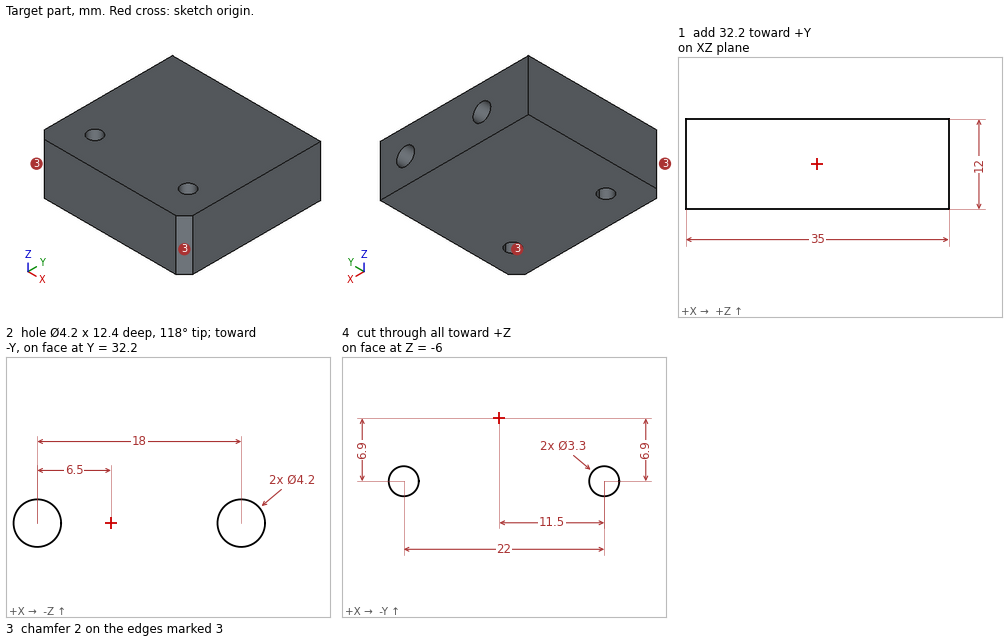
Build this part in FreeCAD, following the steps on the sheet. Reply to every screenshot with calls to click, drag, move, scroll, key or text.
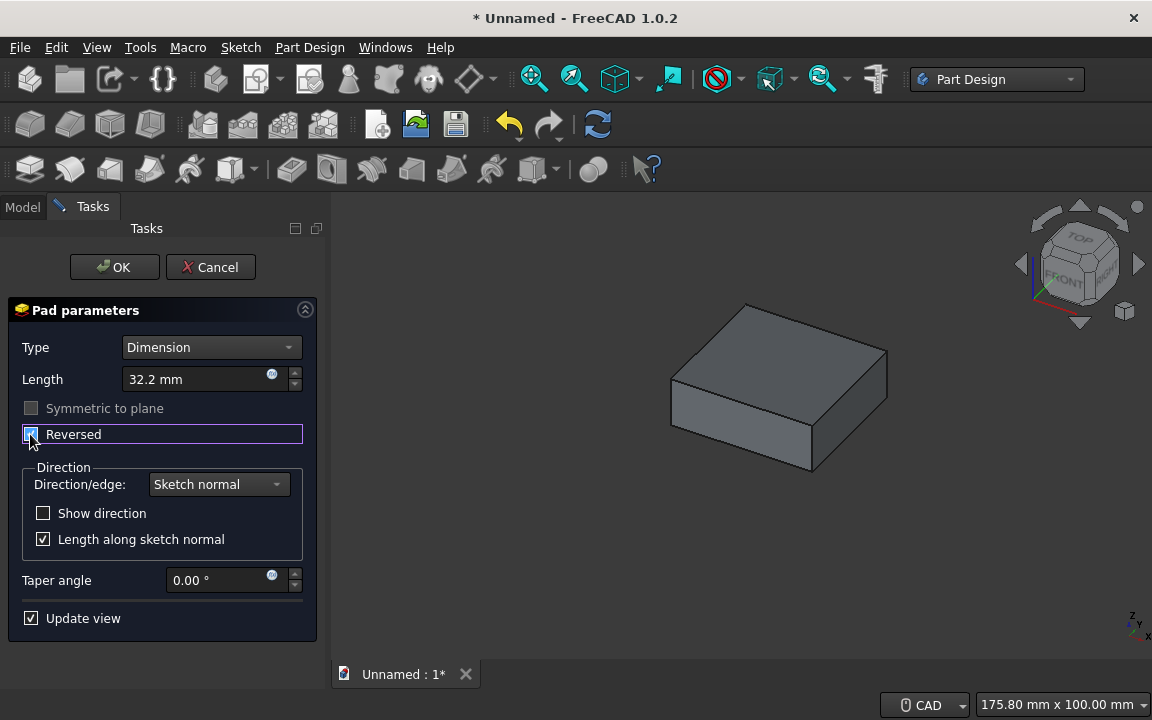
click(115, 267)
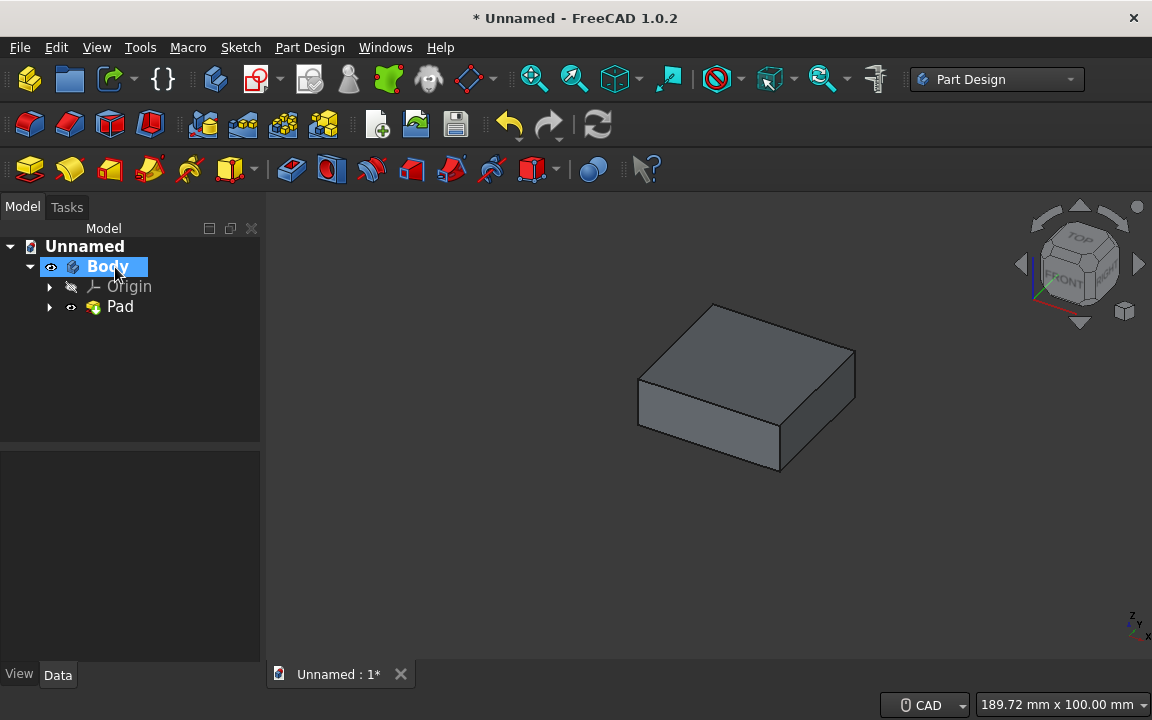
key(v)
key(f)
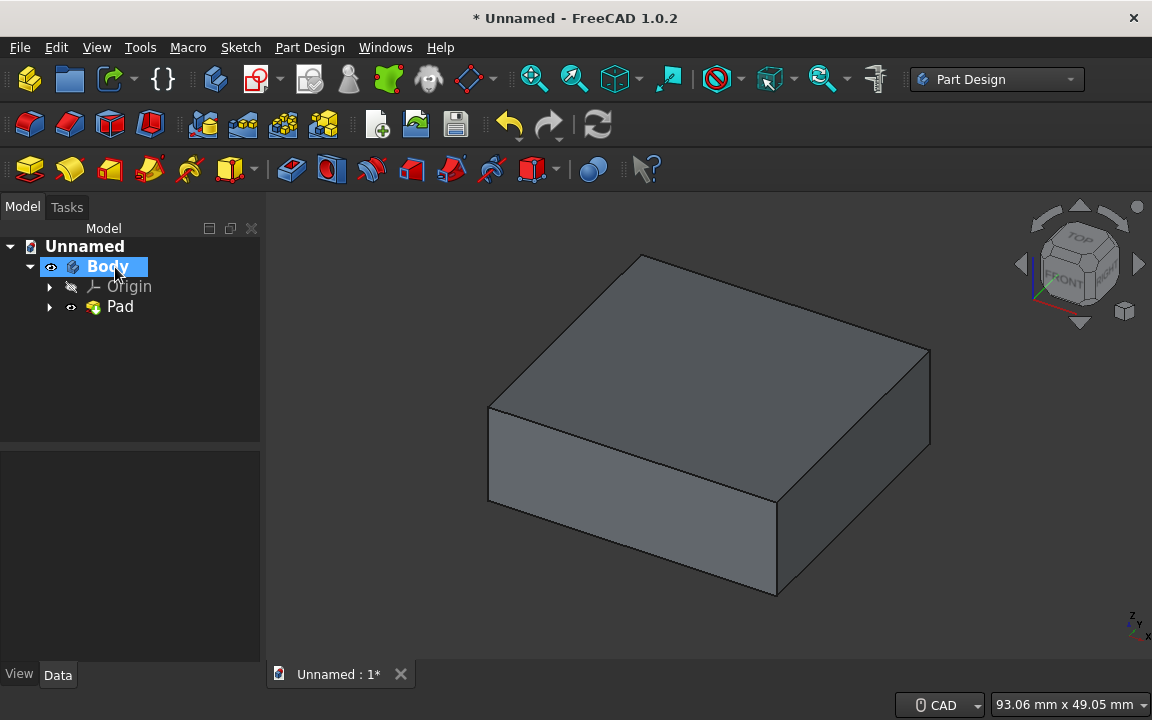
key(4)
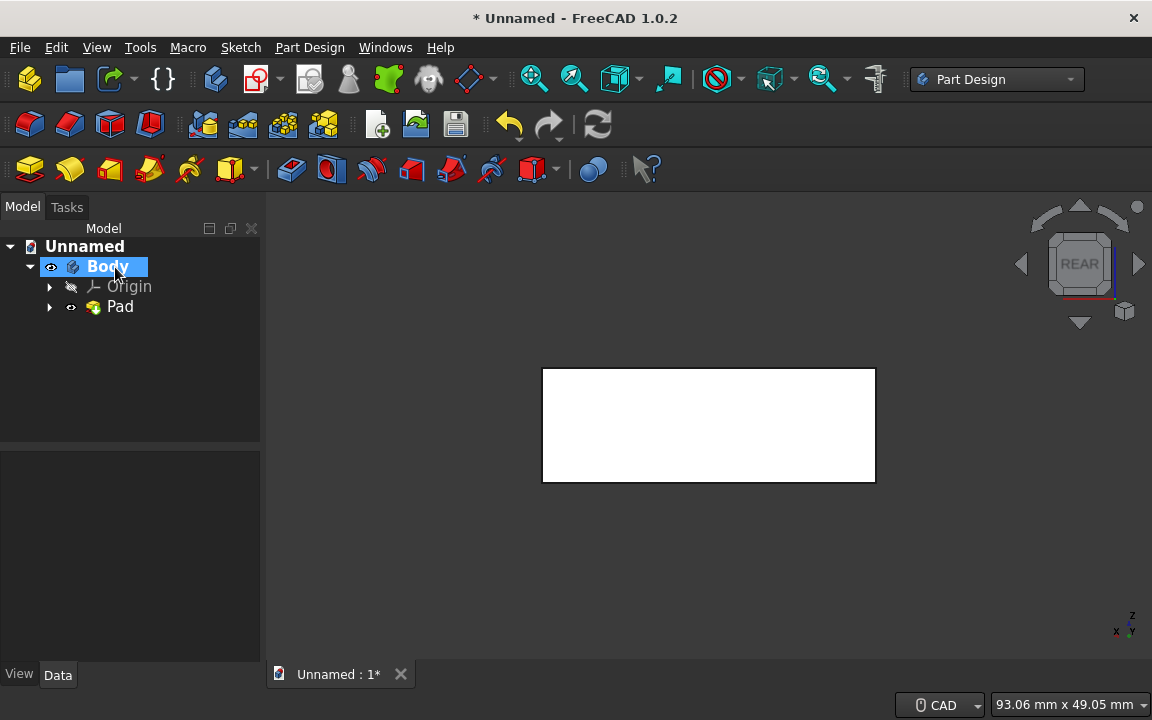
click(536, 80)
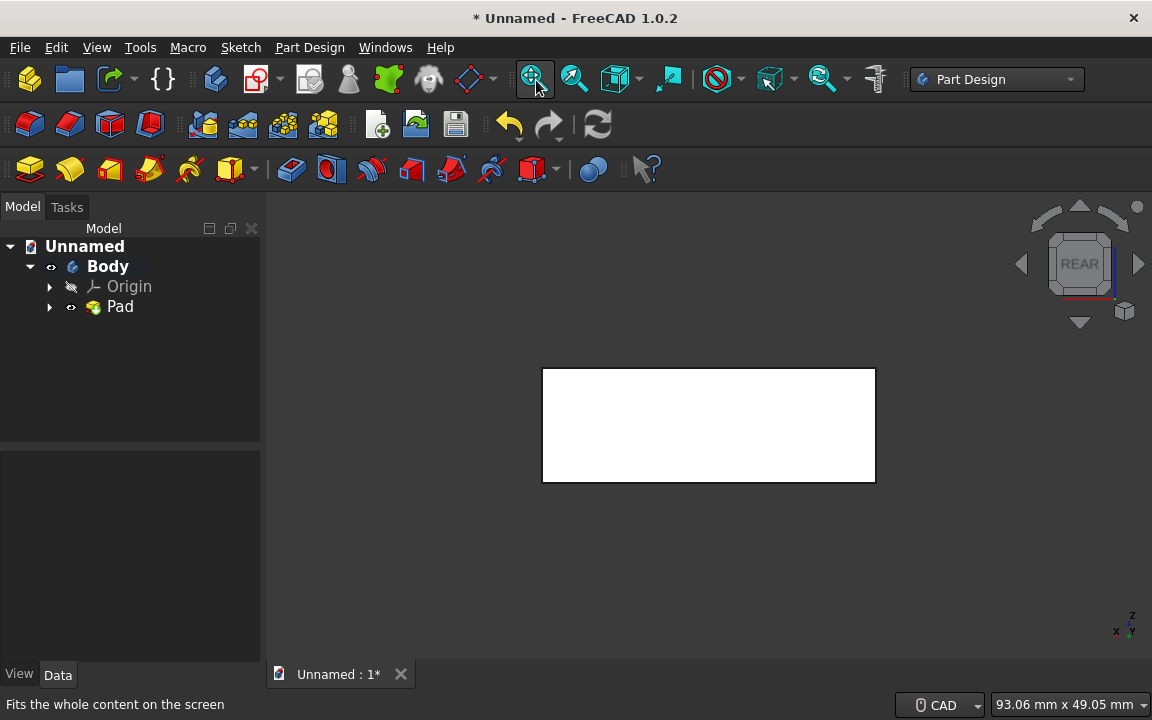
click(614, 425)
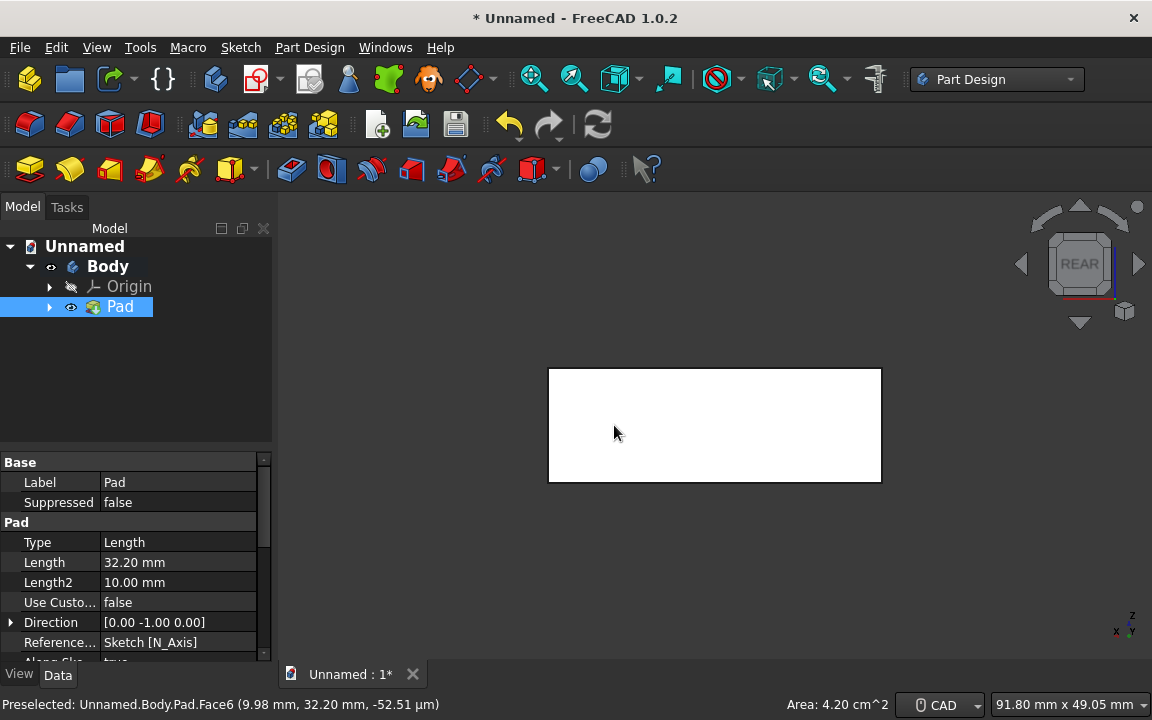
click(256, 80)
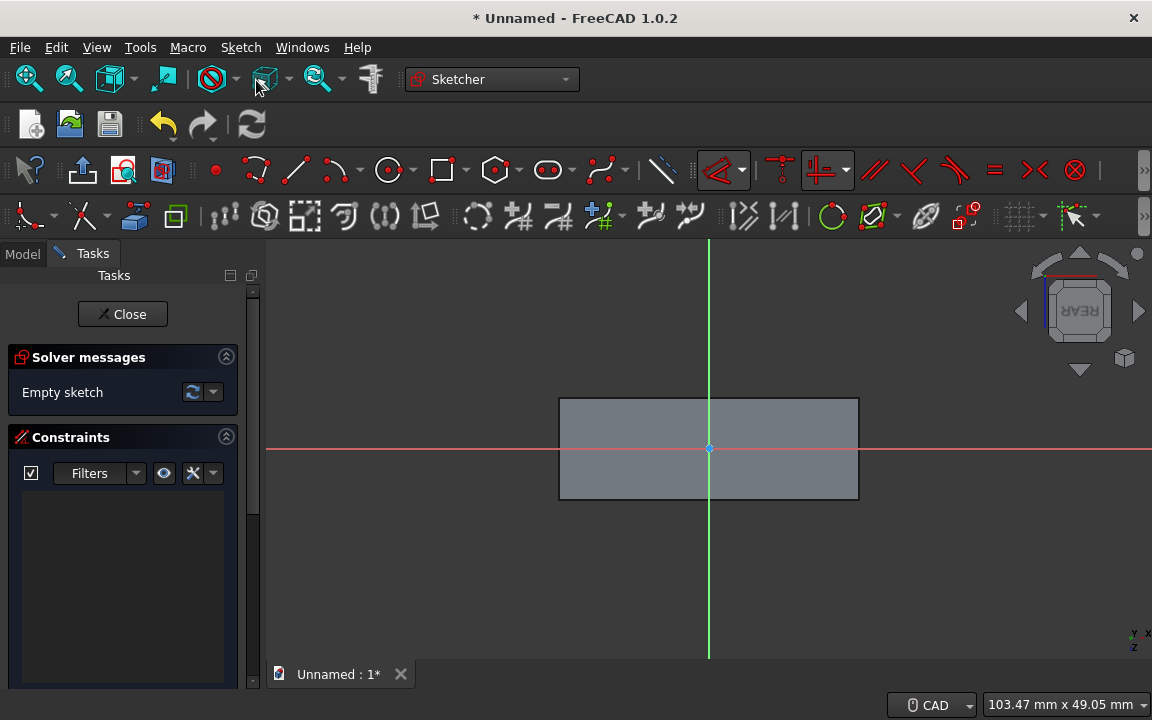
scroll(783, 449, up, 5)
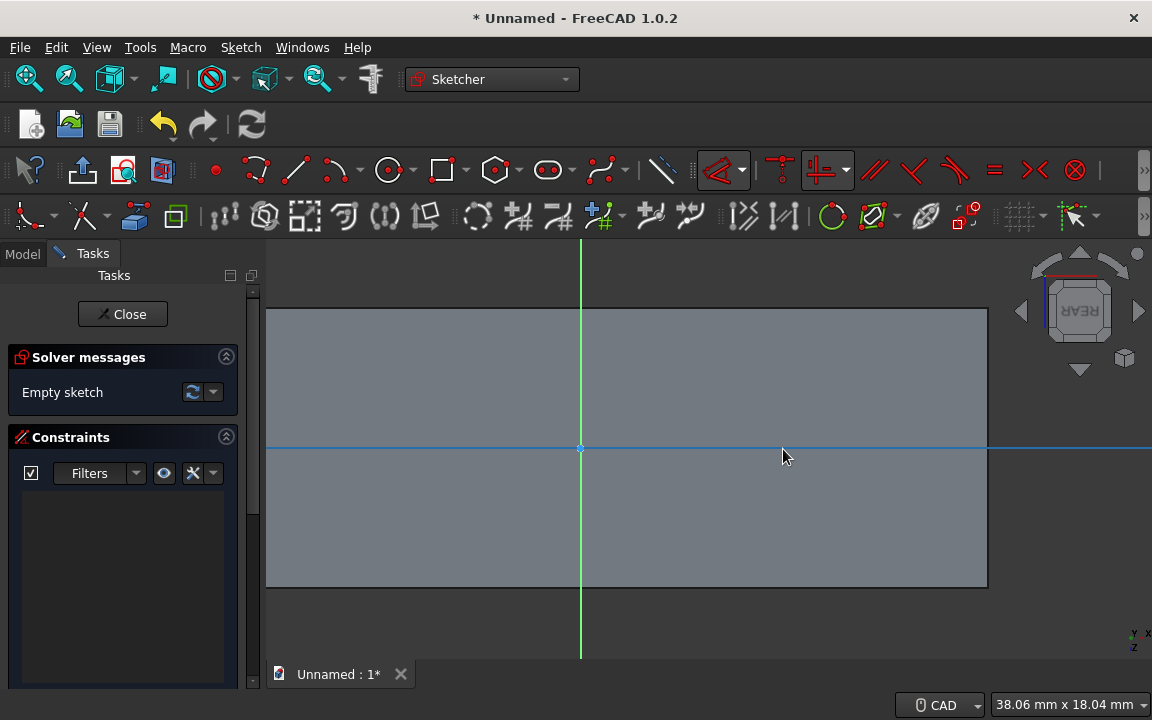
click(390, 170)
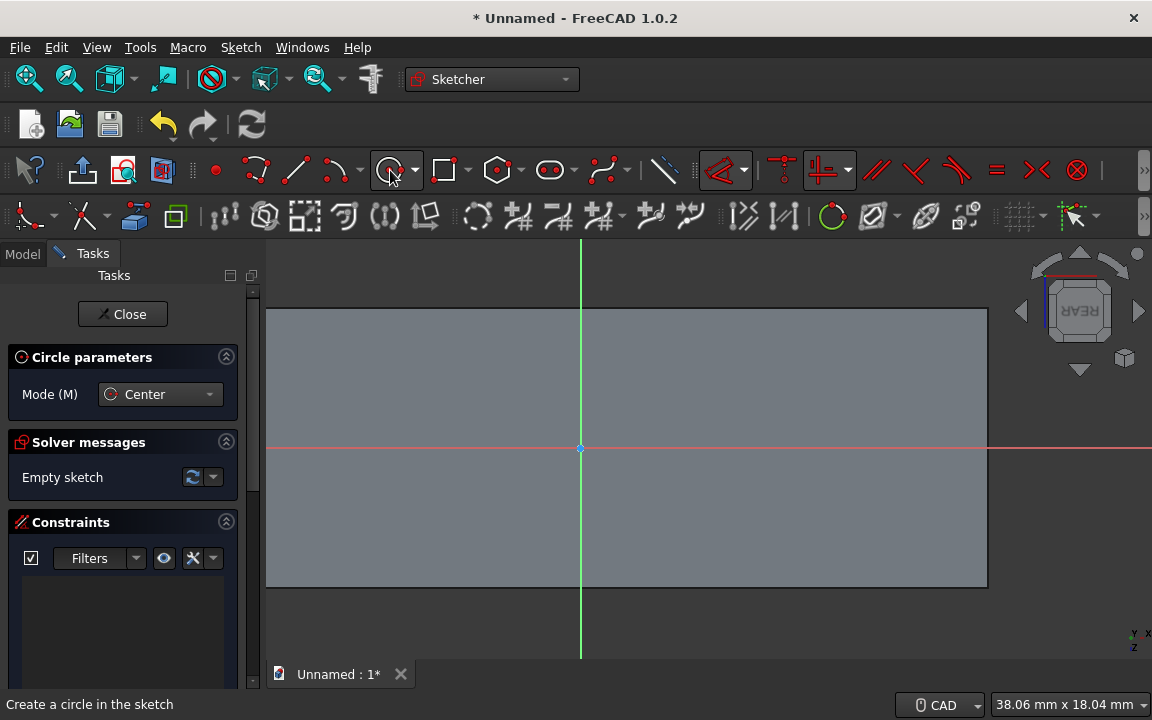
click(849, 448)
move(883, 414)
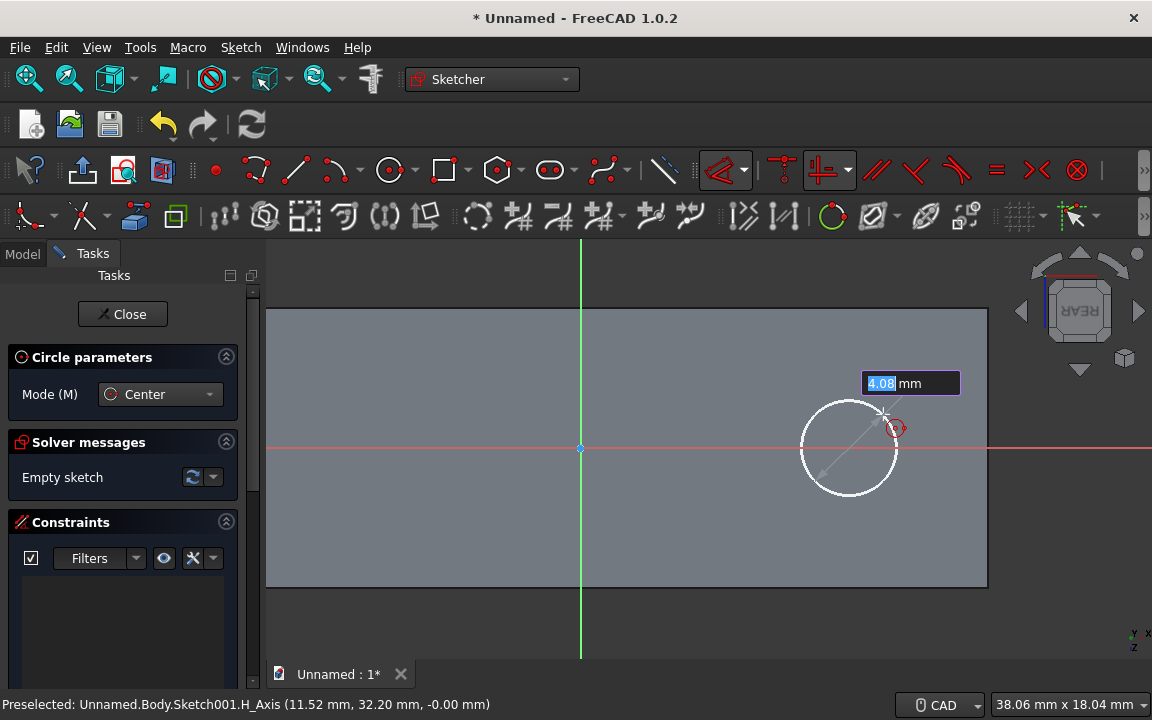
text(4.2)
key(Return)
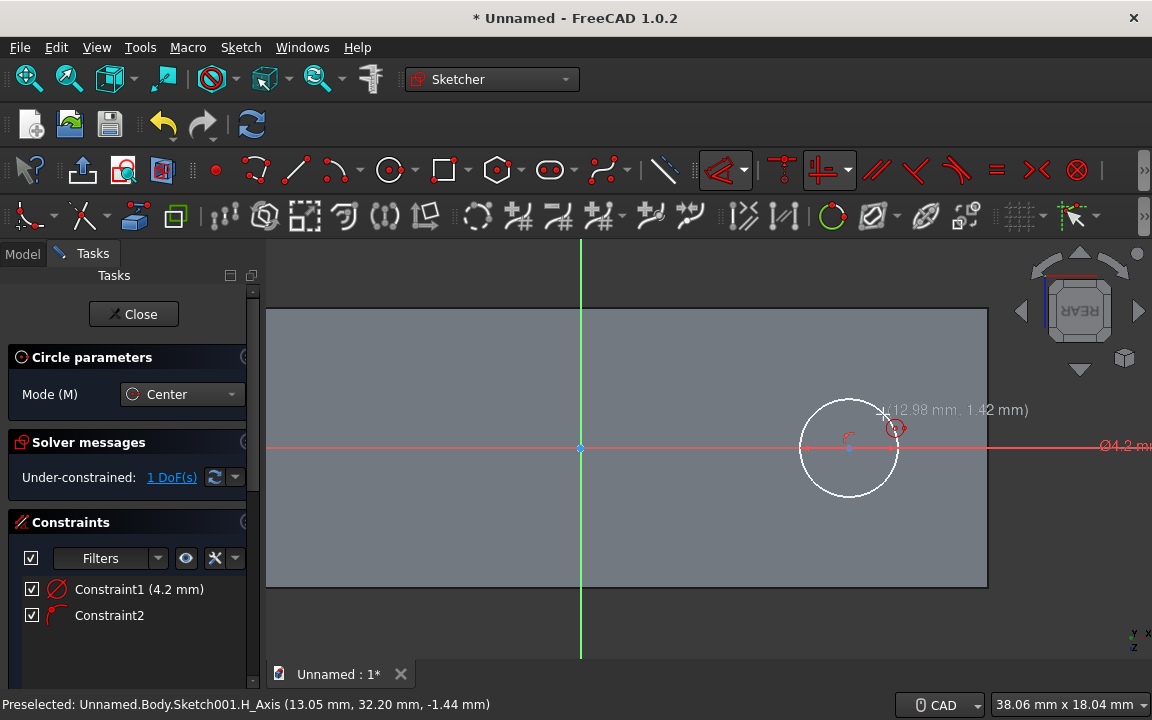
click(430, 448)
move(464, 414)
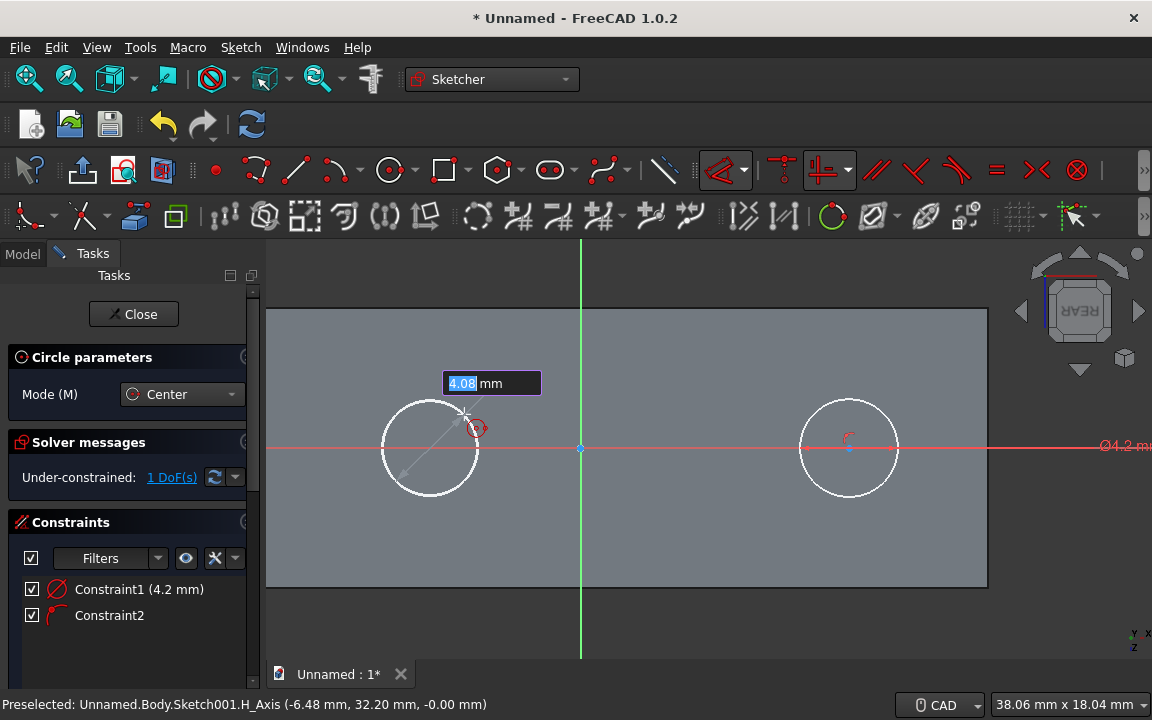
text(4.2)
key(Return)
key(Escape)